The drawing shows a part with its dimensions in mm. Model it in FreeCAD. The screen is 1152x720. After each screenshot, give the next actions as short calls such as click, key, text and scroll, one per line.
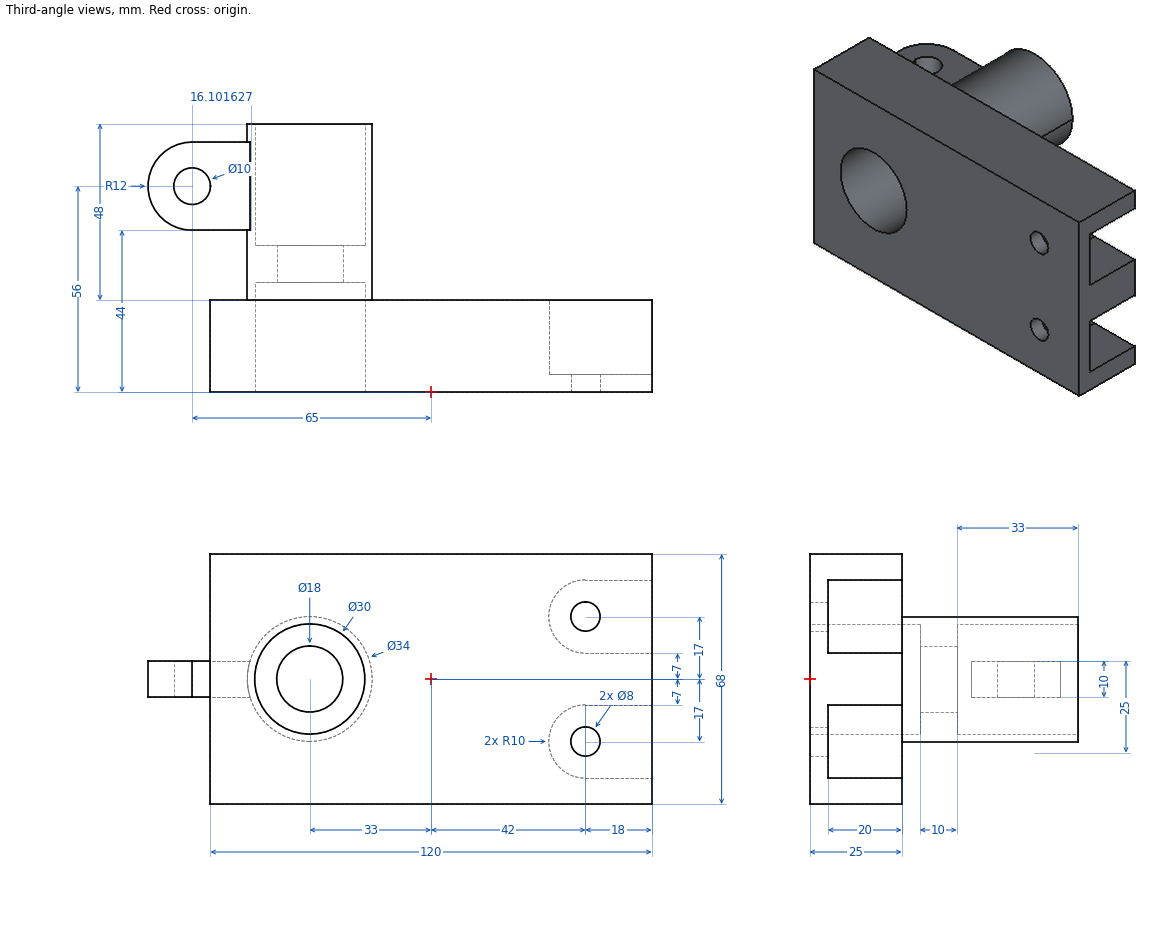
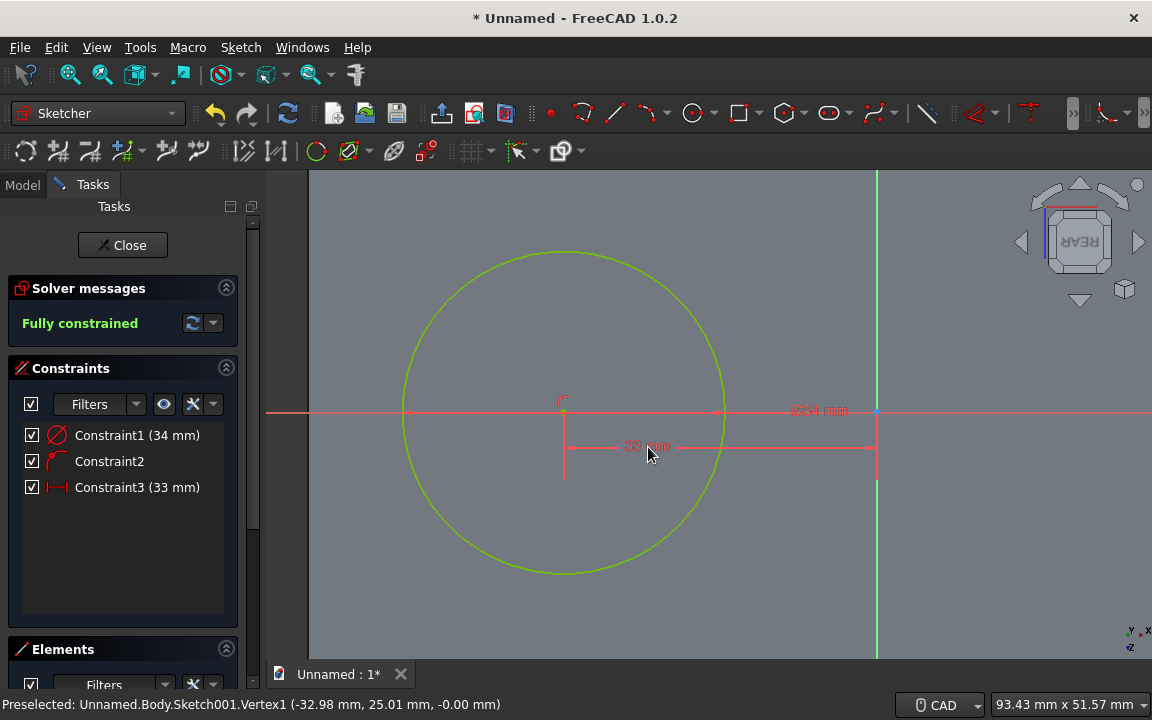
click(123, 245)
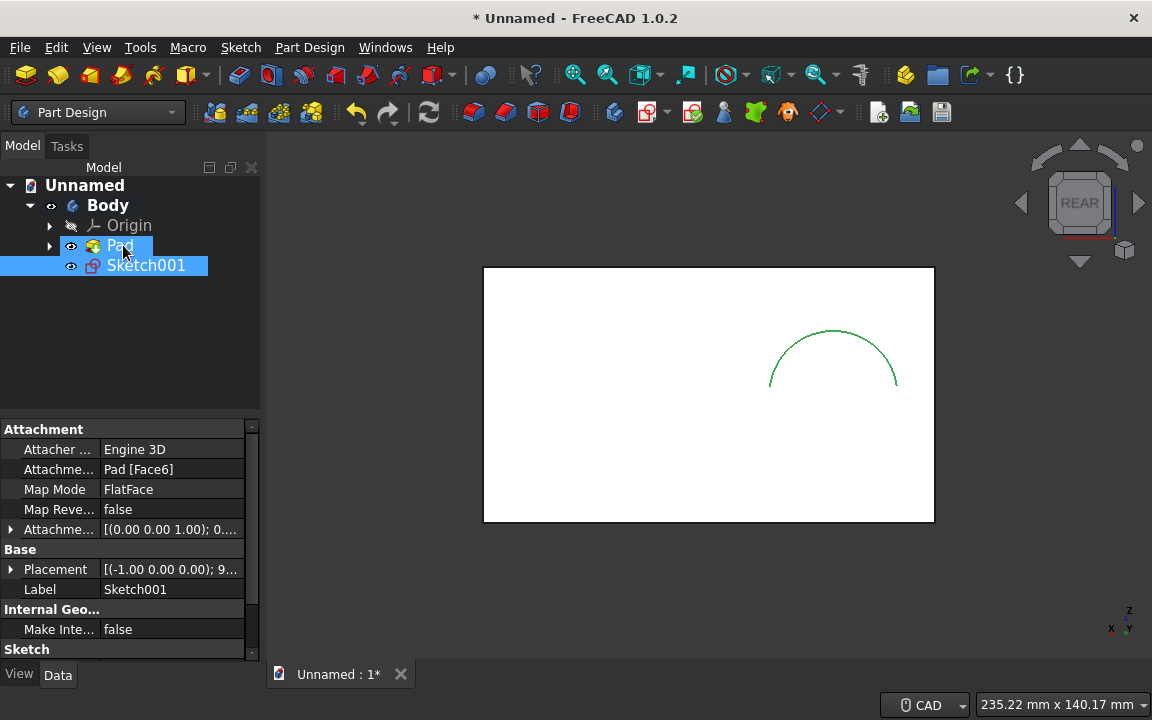
click(26, 76)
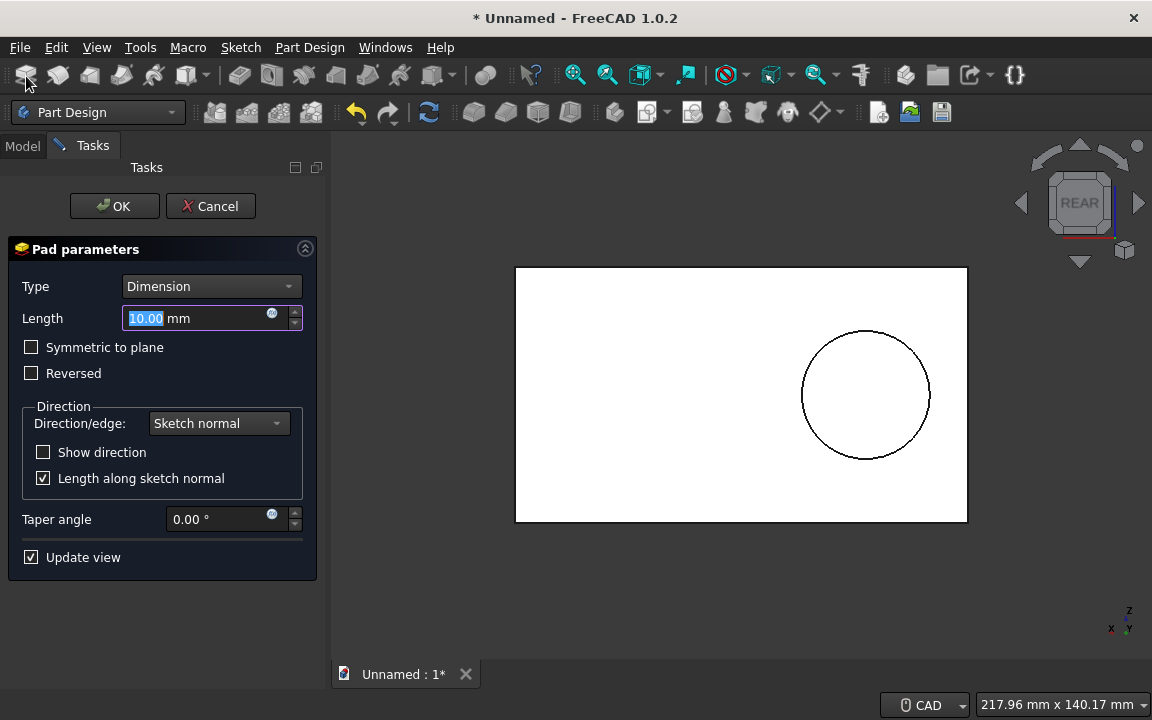
text(48)
key(Tab)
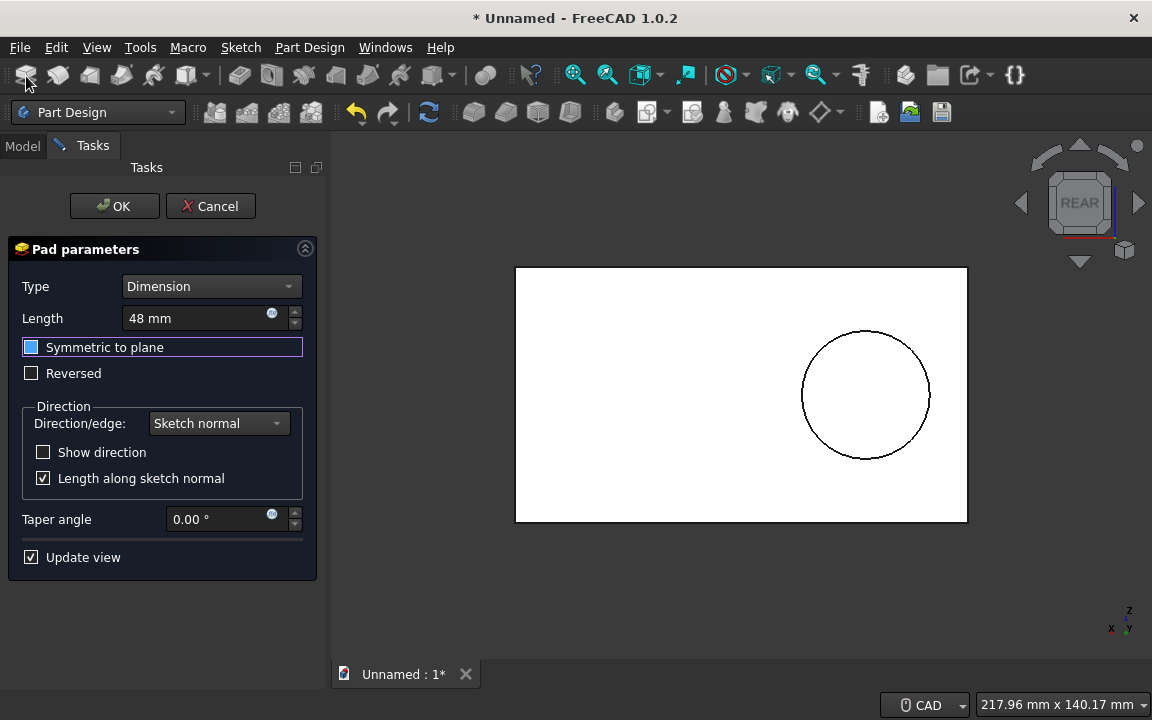
click(115, 206)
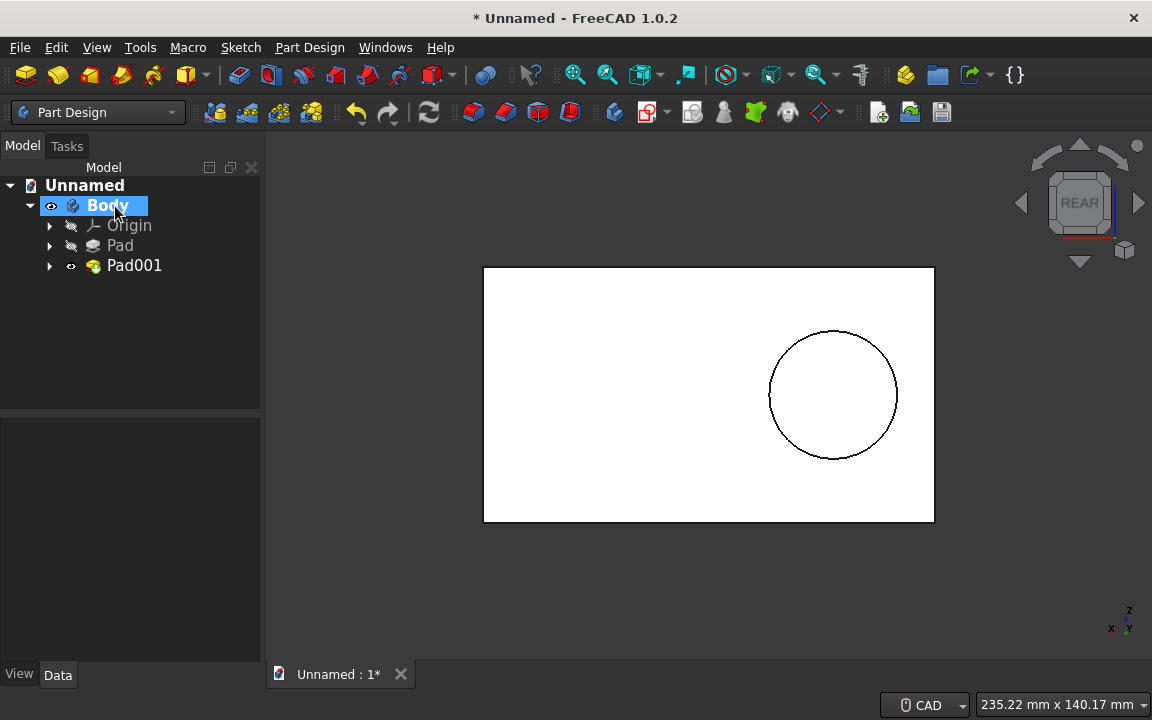
click(648, 112)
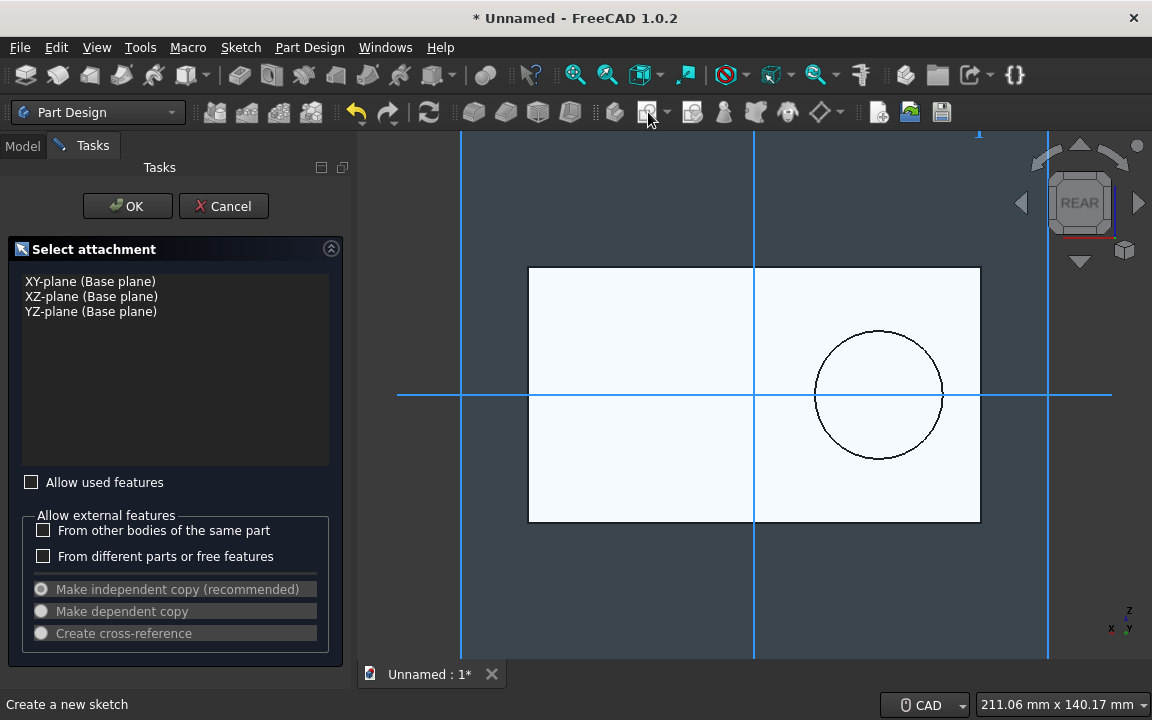
click(82, 282)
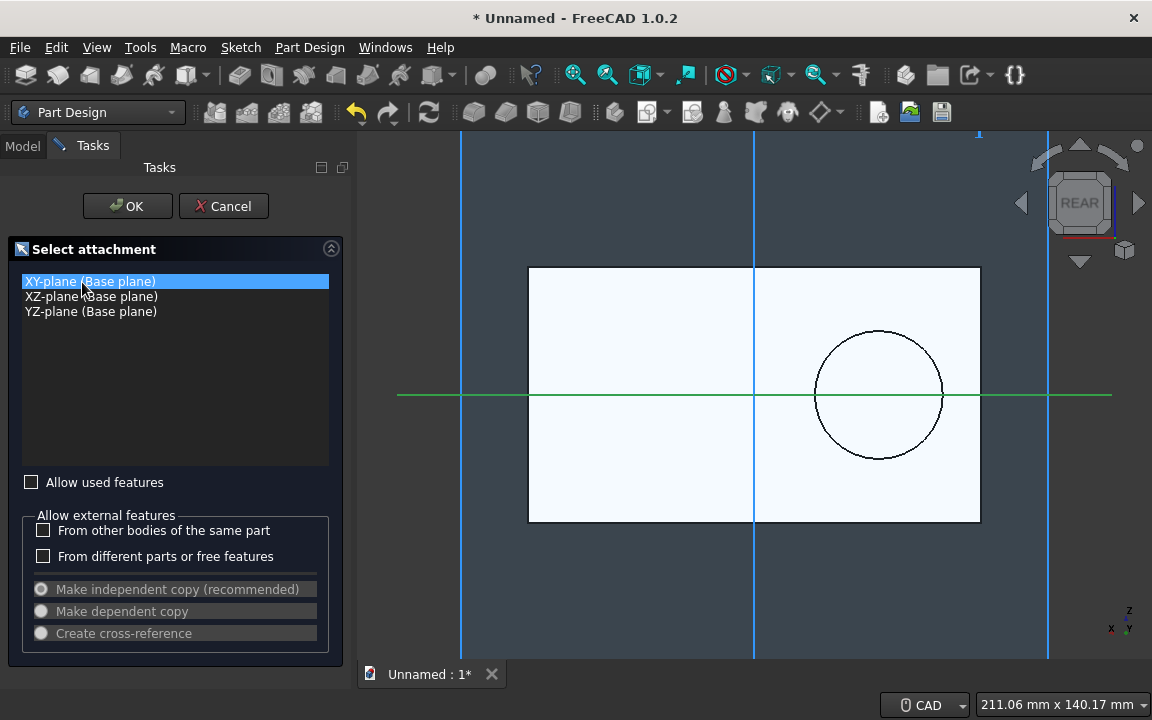
click(128, 206)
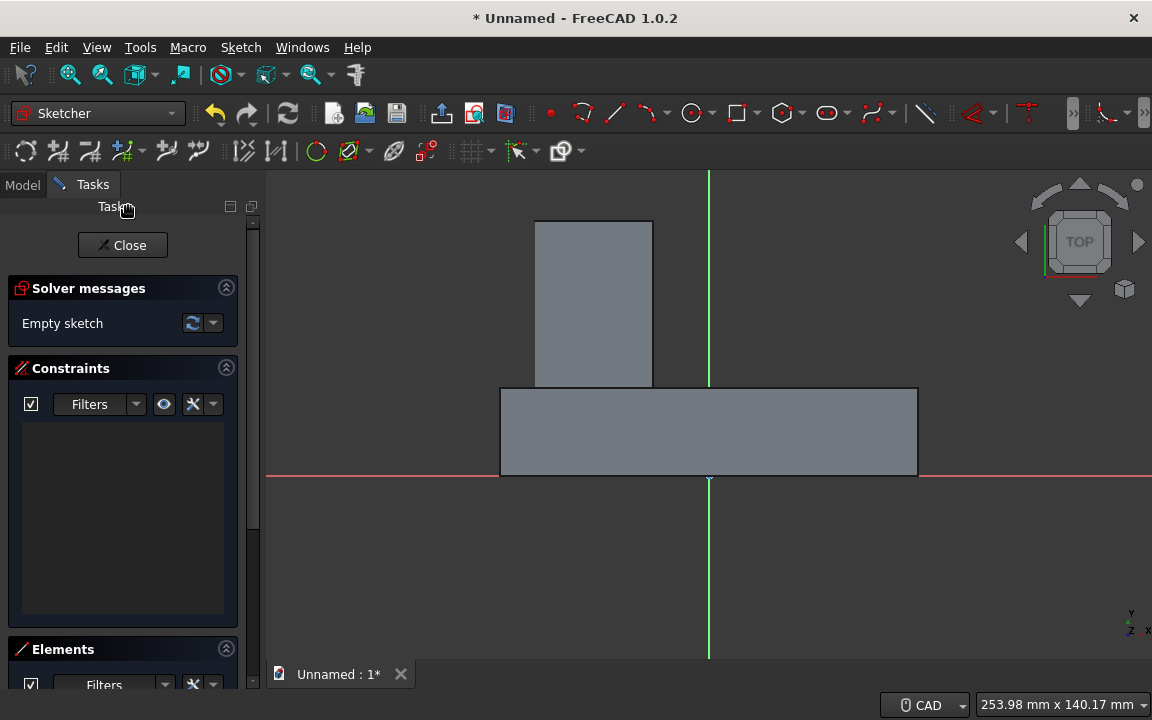
click(506, 114)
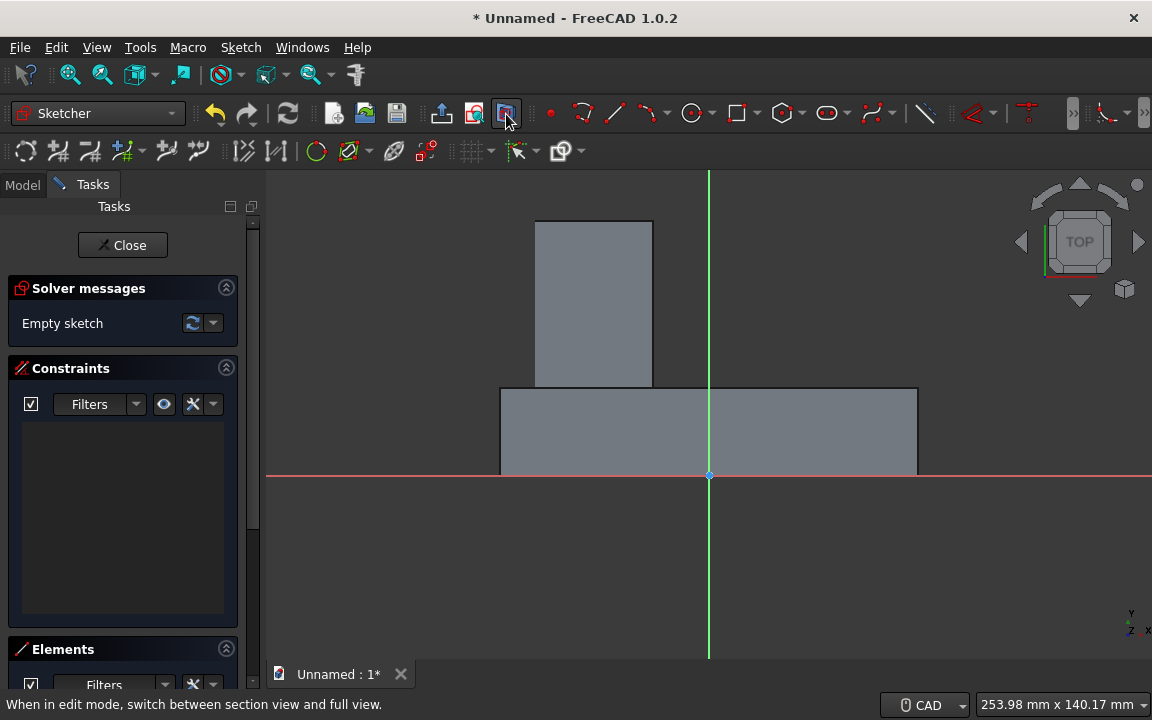
scroll(424, 222, up, 6)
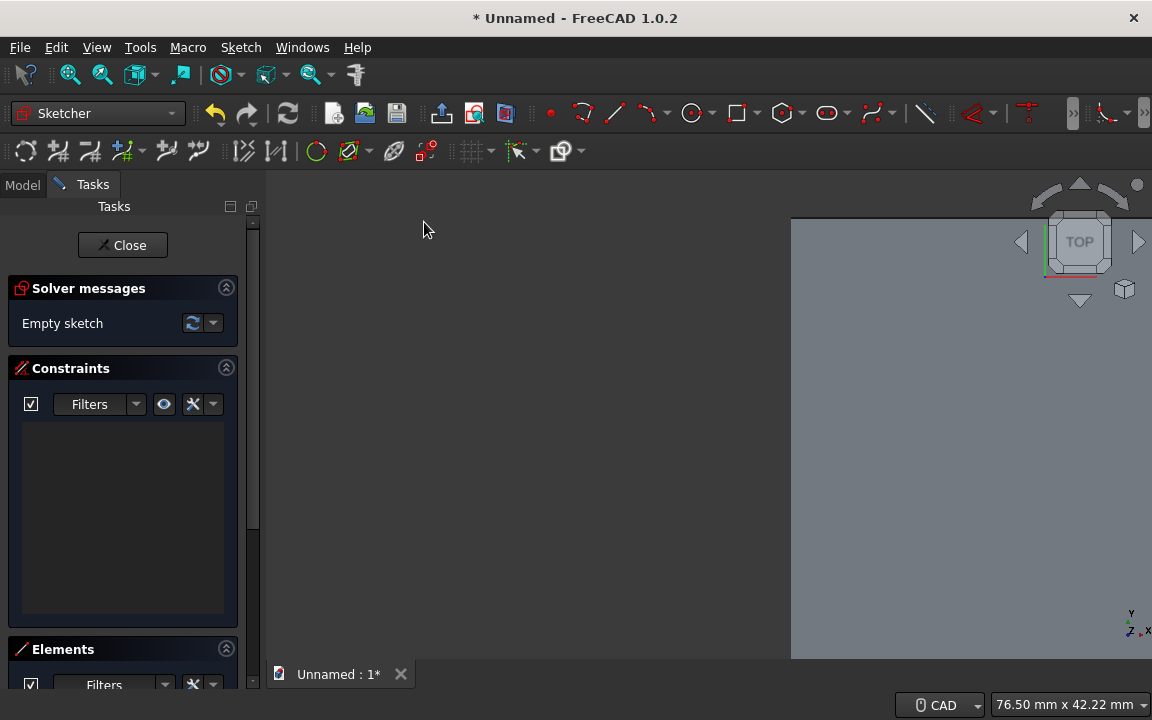
click(584, 114)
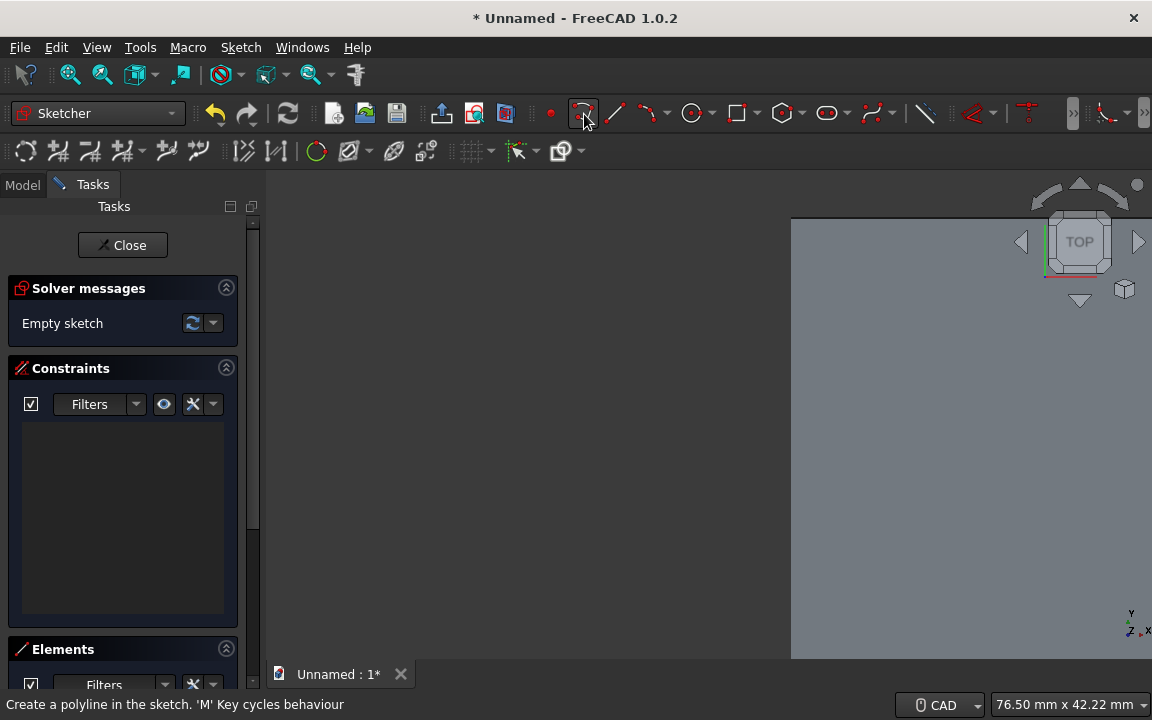
click(617, 554)
click(803, 554)
click(803, 276)
click(617, 276)
right_click(617, 276)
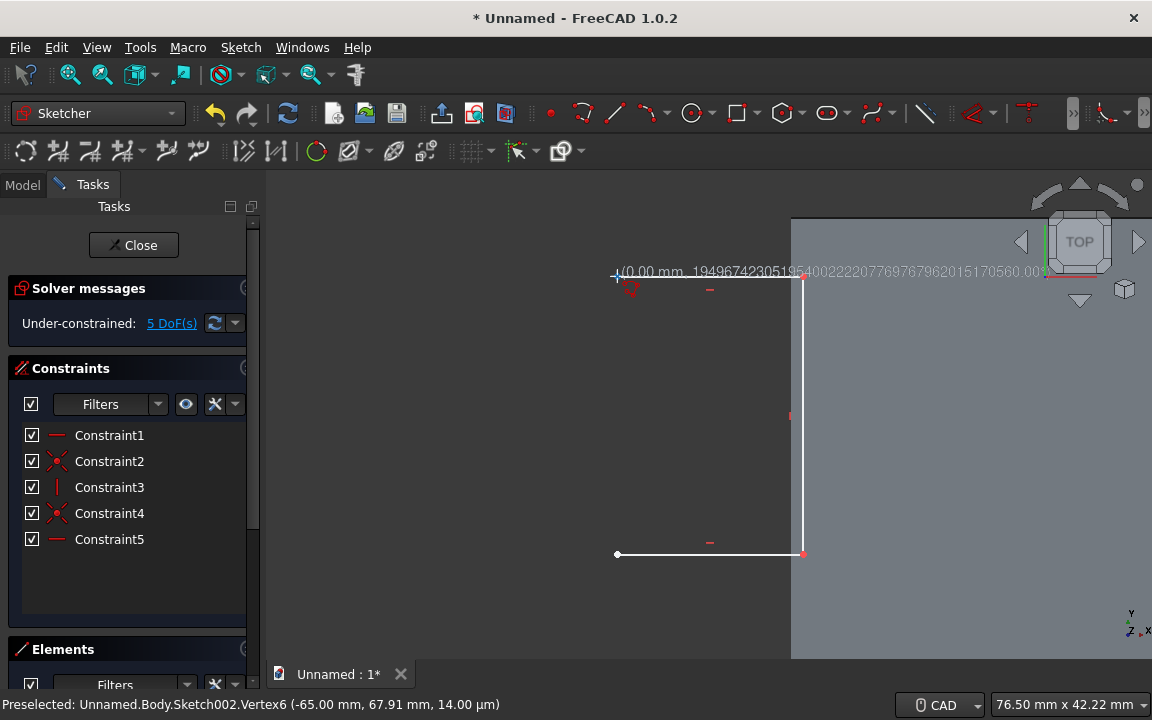
click(648, 114)